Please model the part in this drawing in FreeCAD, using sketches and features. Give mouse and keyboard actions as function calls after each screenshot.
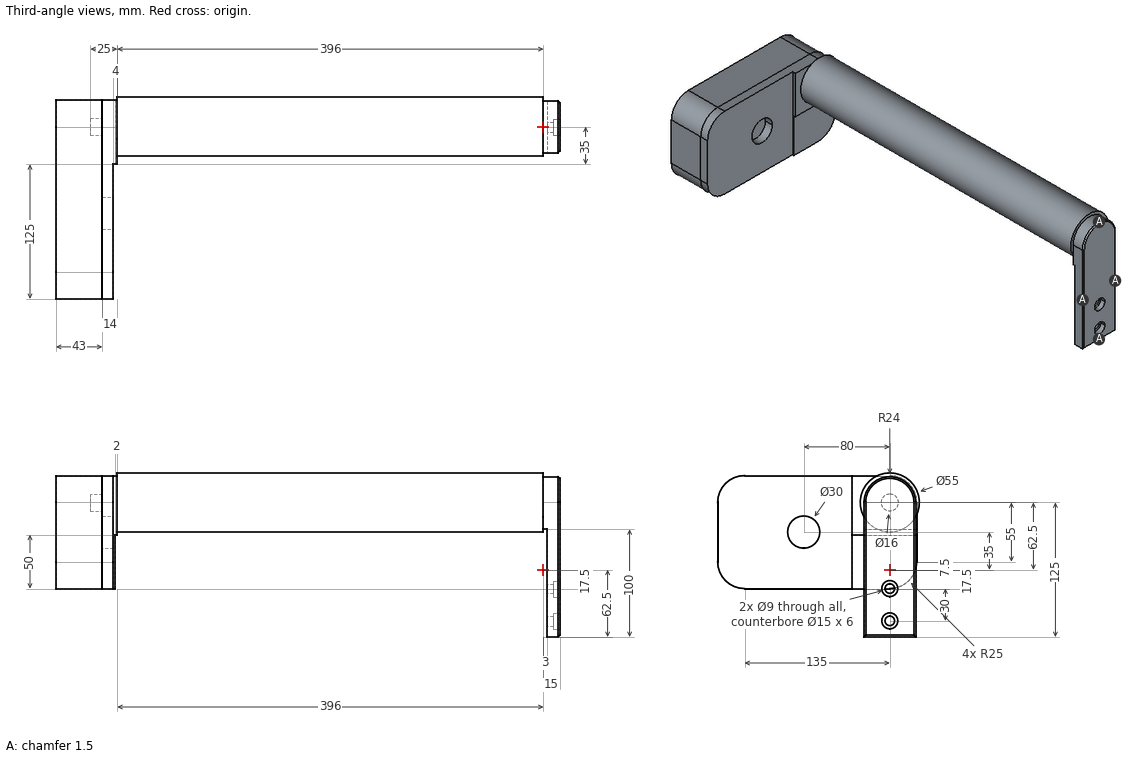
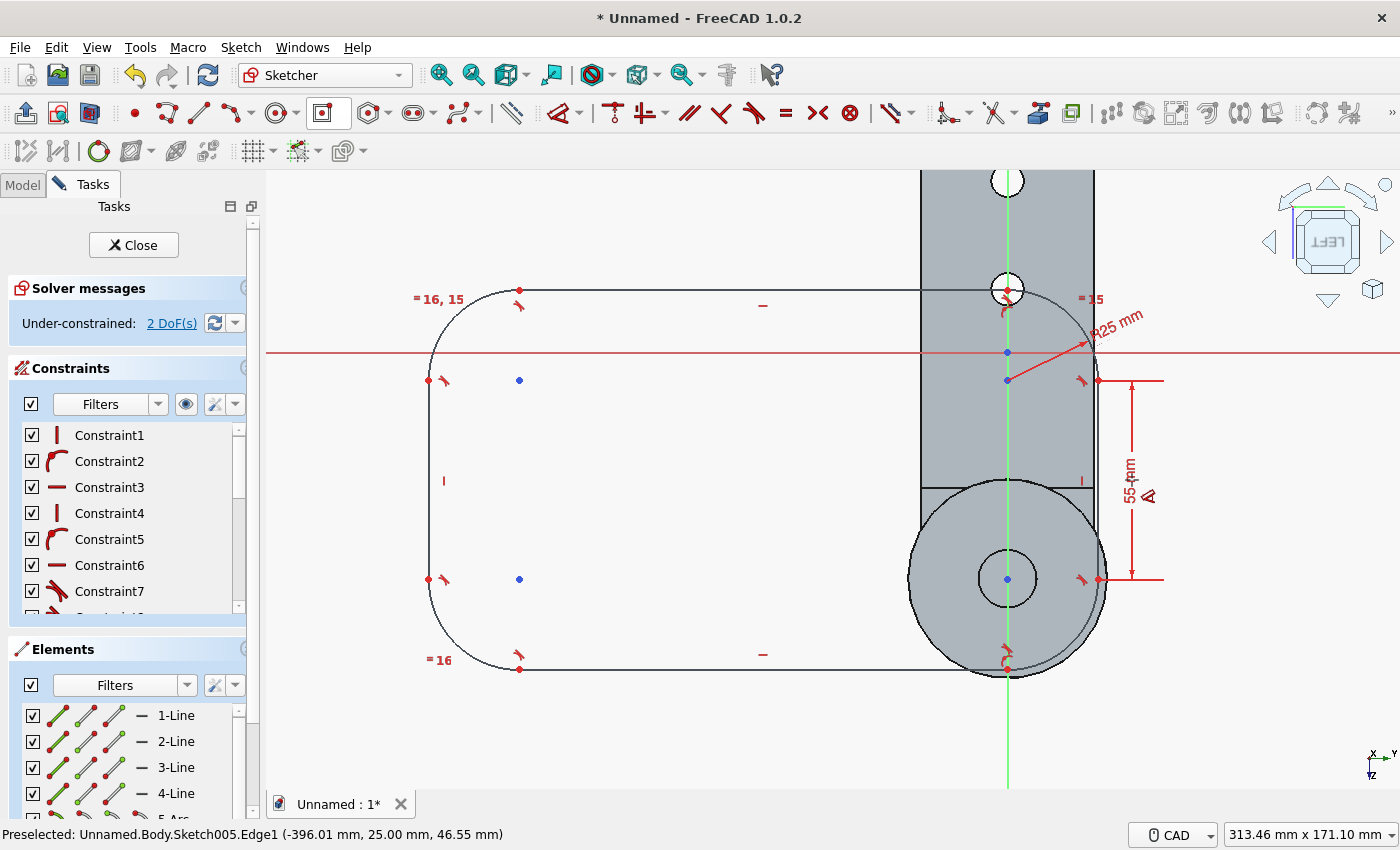
click(861, 290)
click(763, 256)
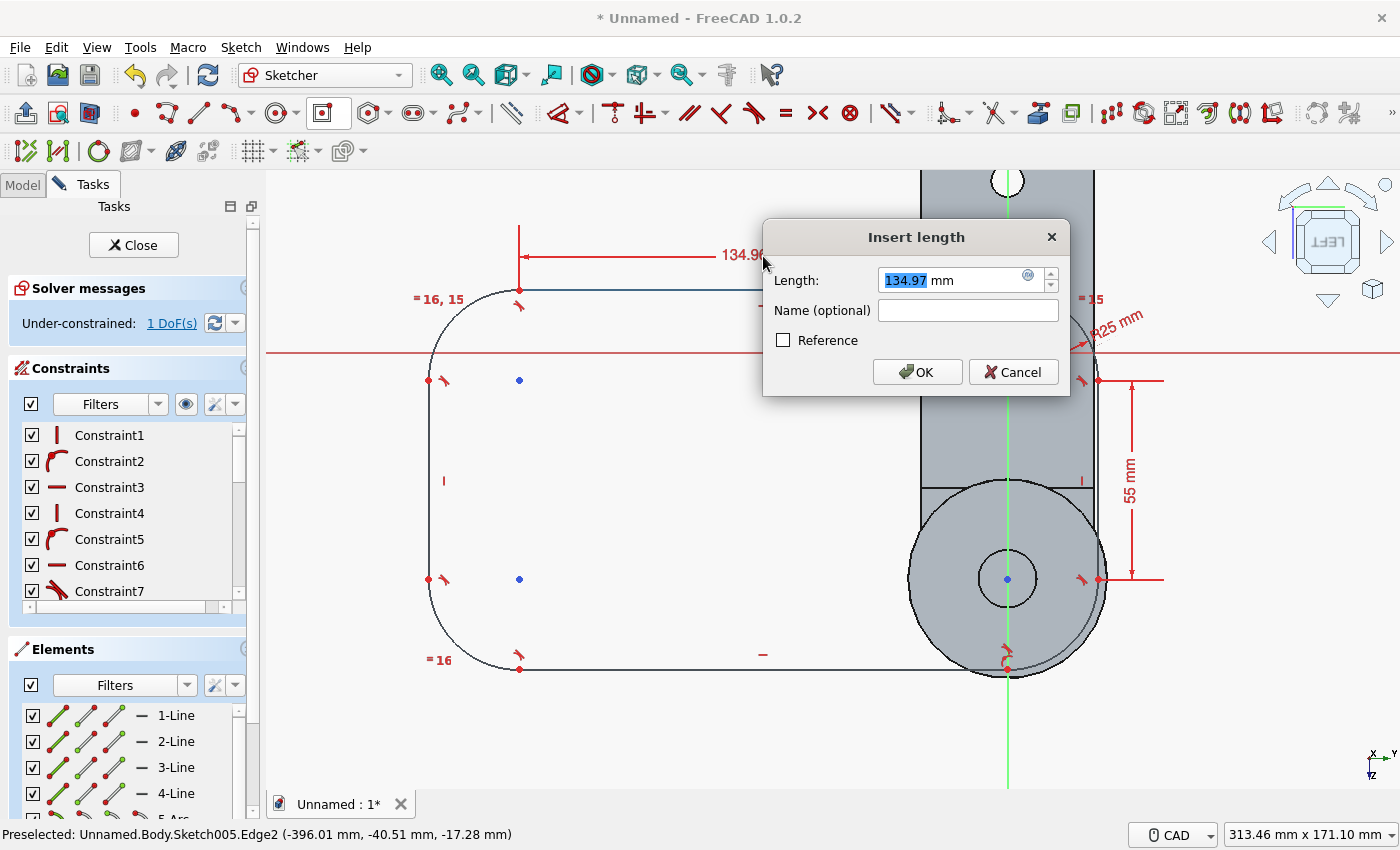
text(135)
key(Return)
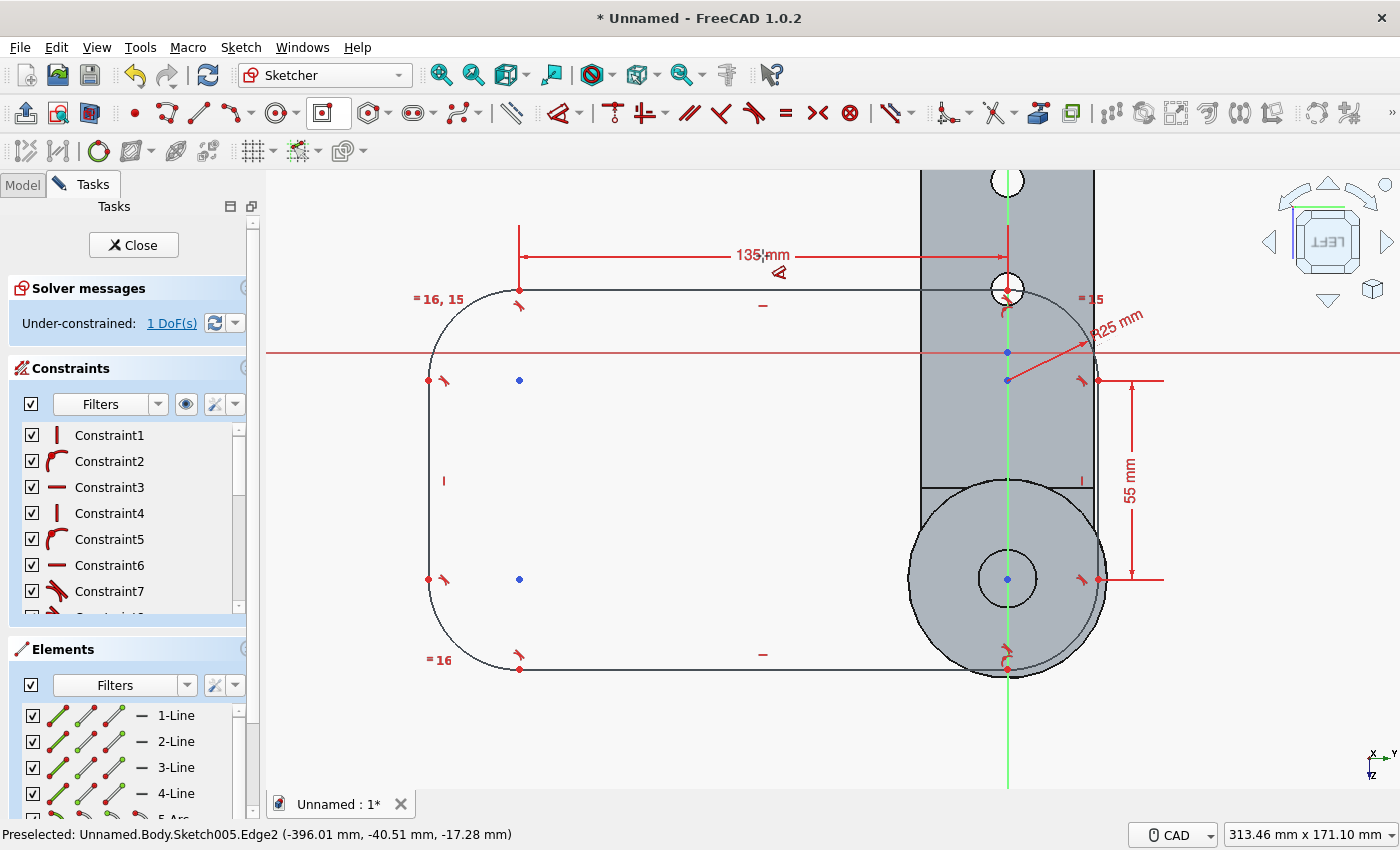
scroll(1098, 381, up, 2)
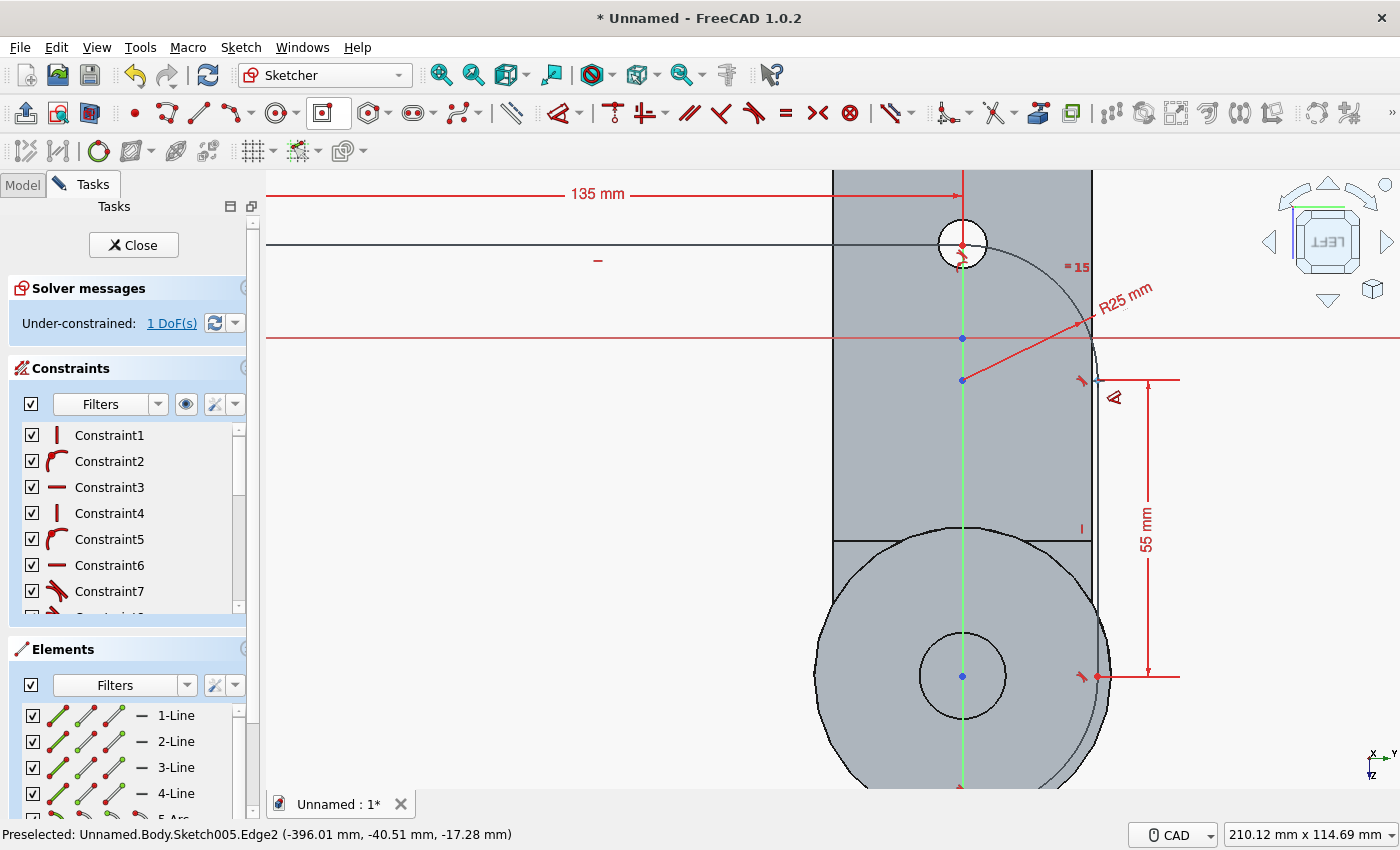
click(1098, 380)
click(1132, 359)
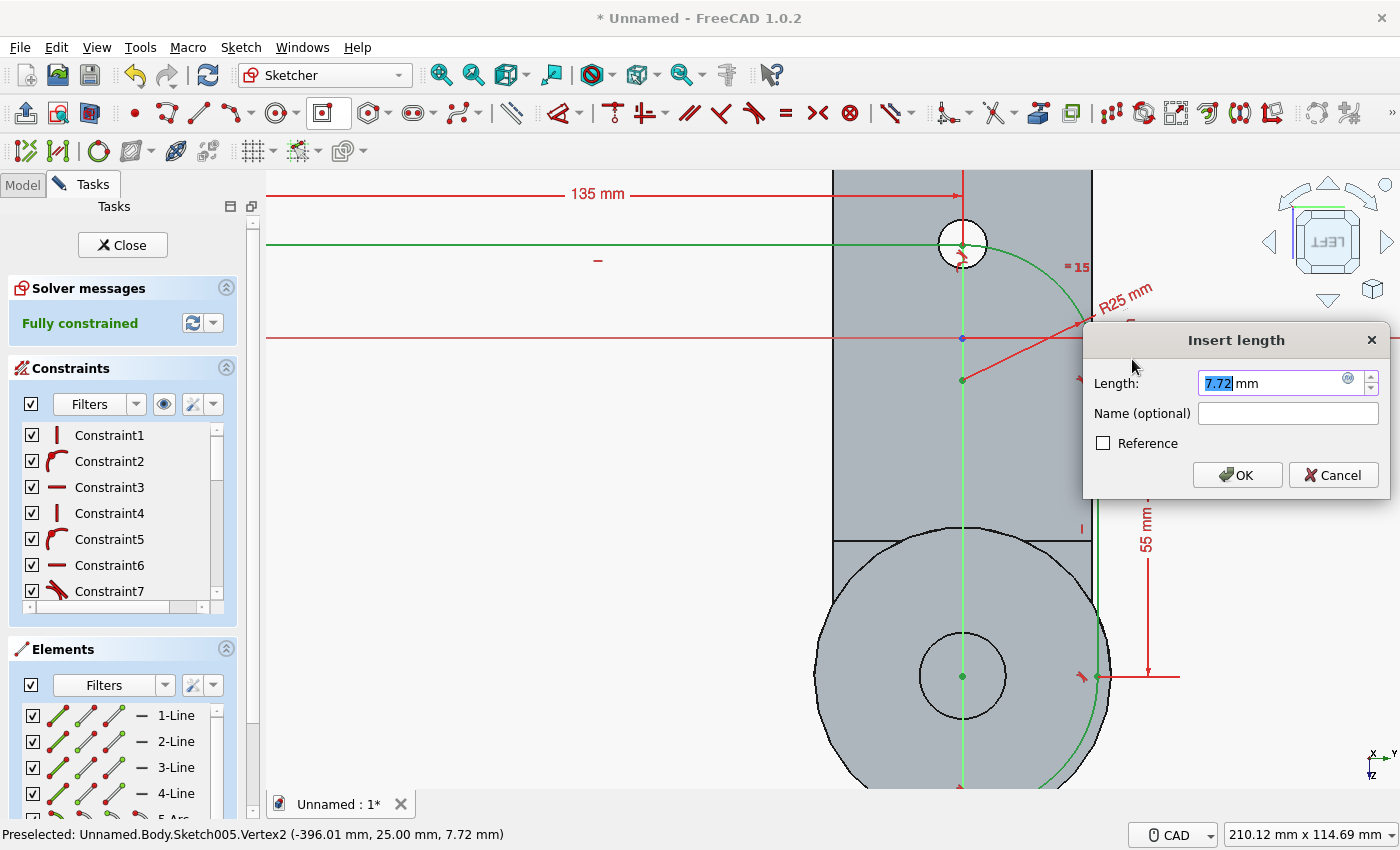
text(7.5)
key(Return)
key(Escape)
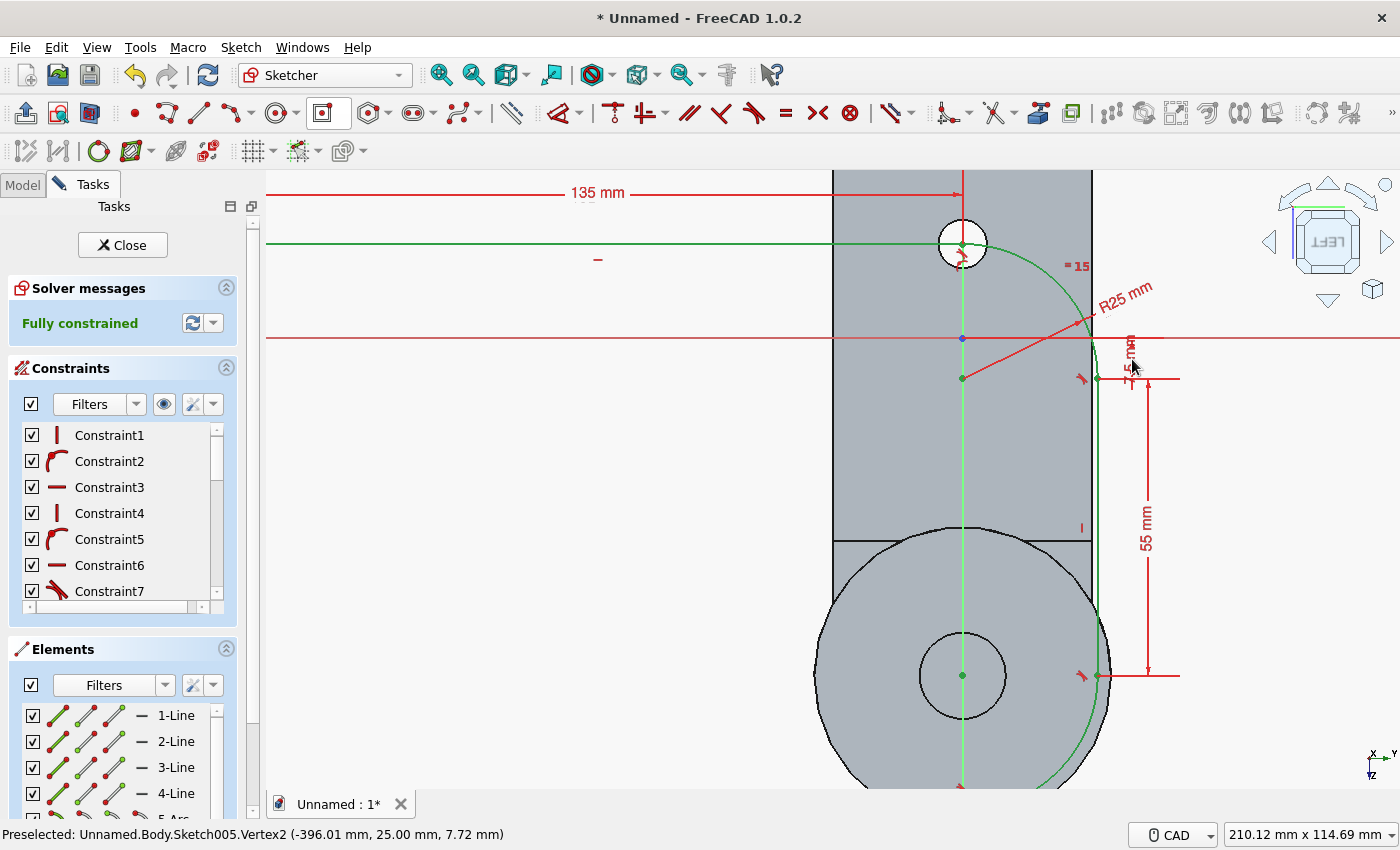
click(123, 245)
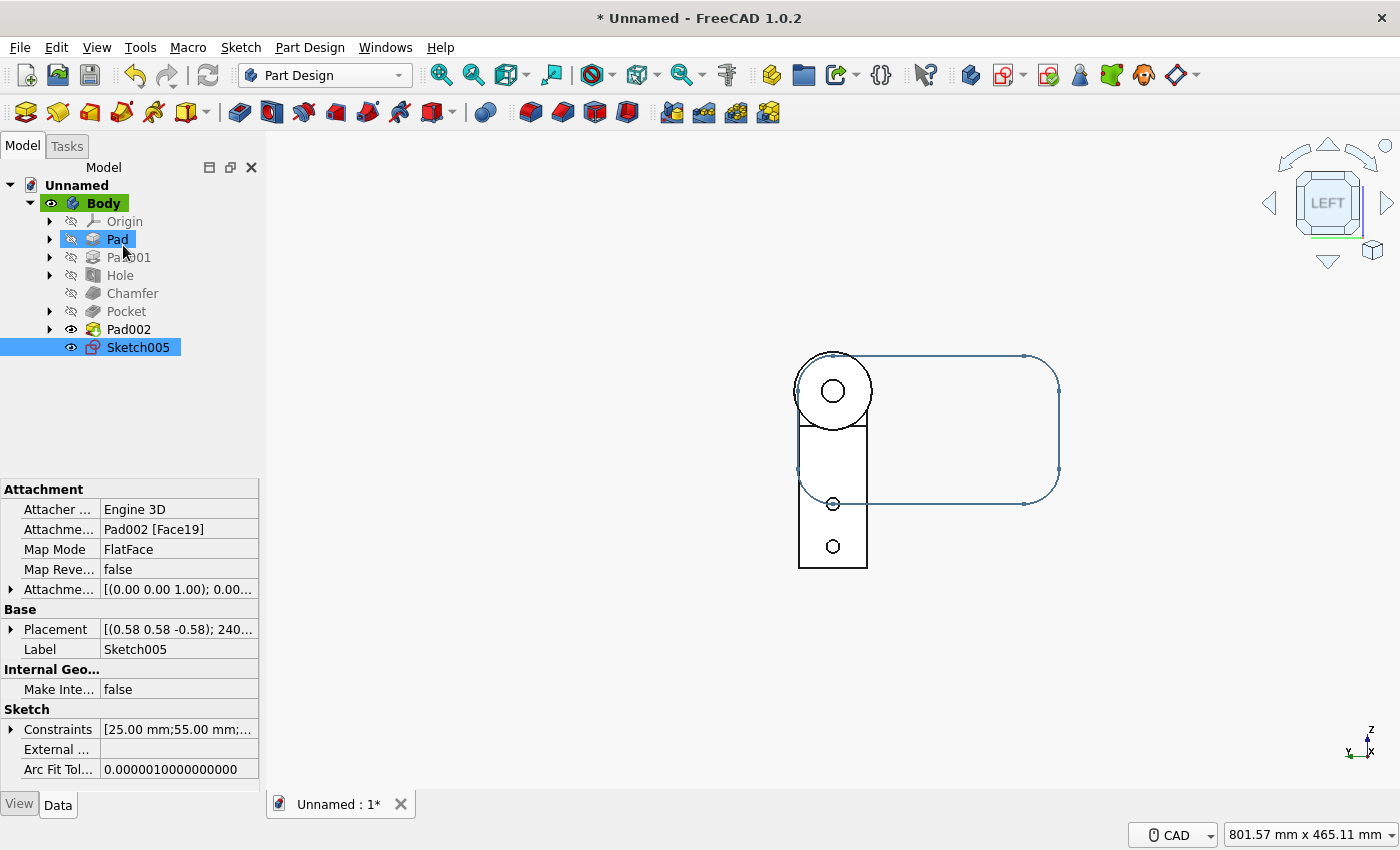
click(26, 112)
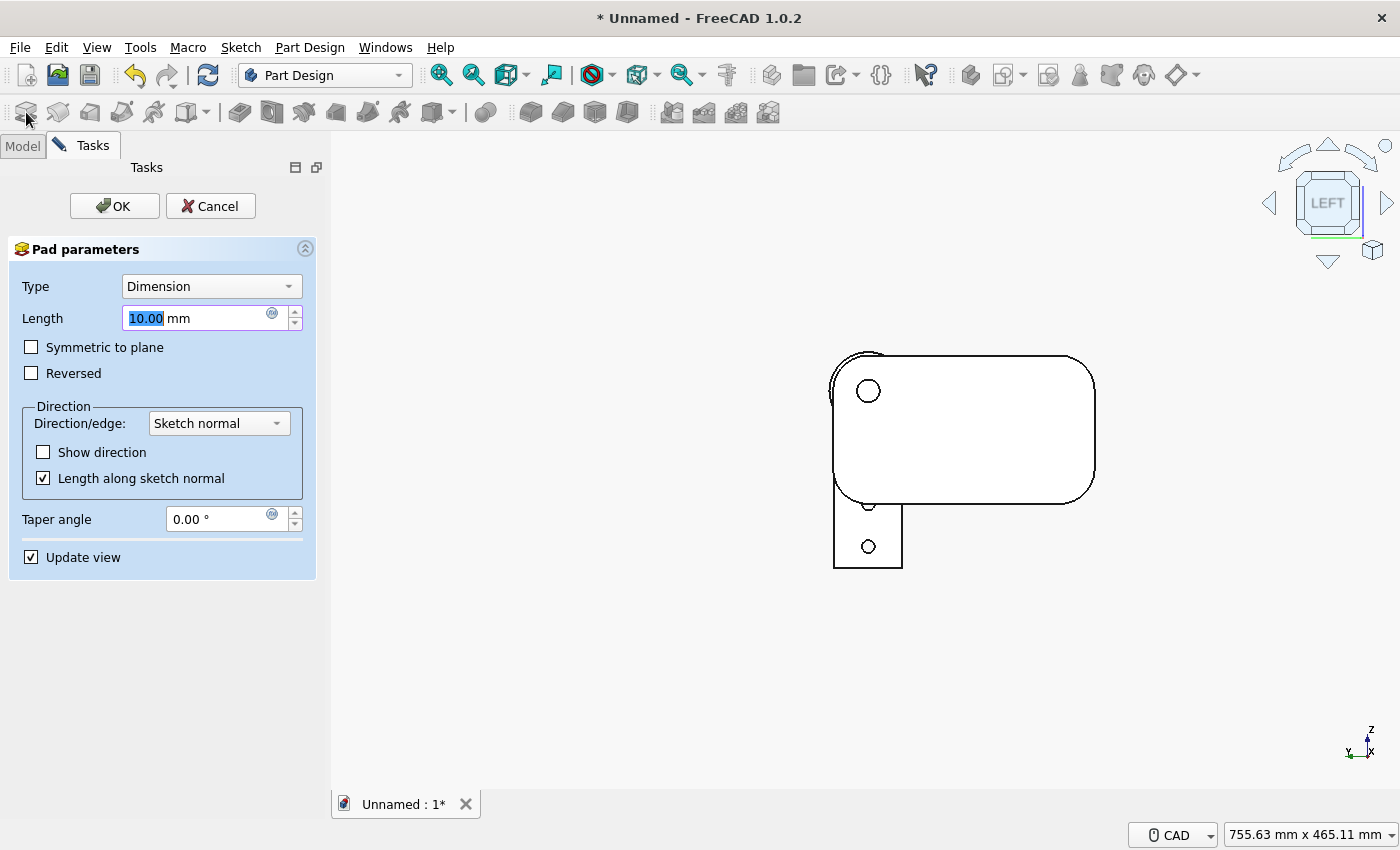
text(14)
key(Tab)